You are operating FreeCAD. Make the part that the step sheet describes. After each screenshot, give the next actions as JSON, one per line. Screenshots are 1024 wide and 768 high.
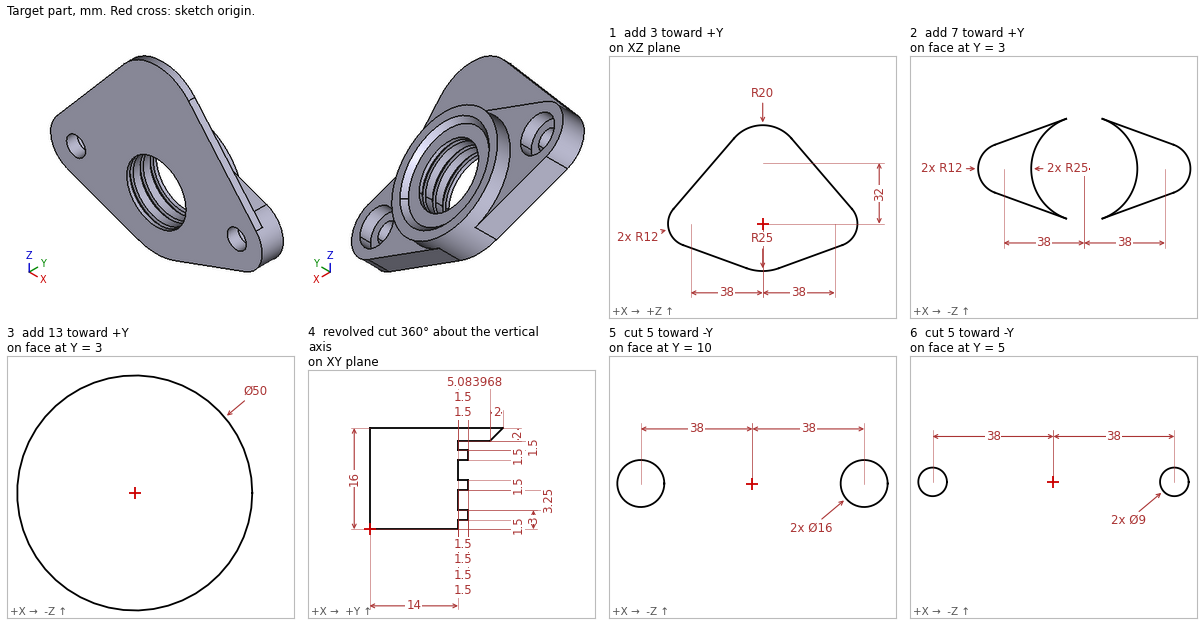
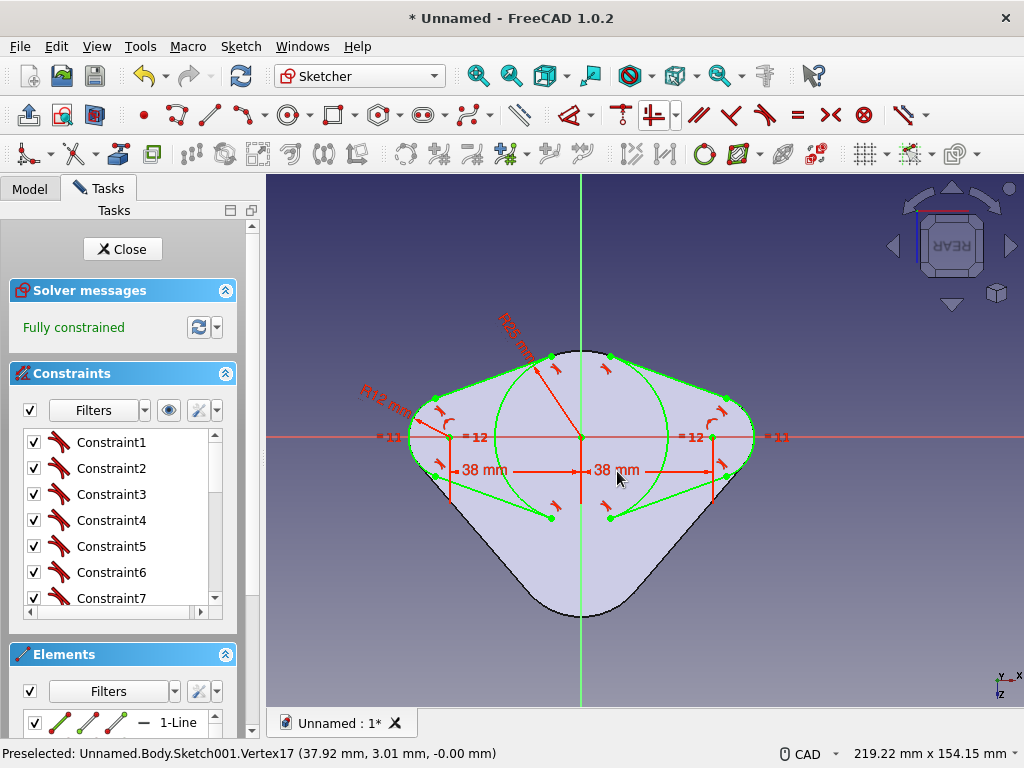
{"action": "left_click", "coordinate": [123, 249]}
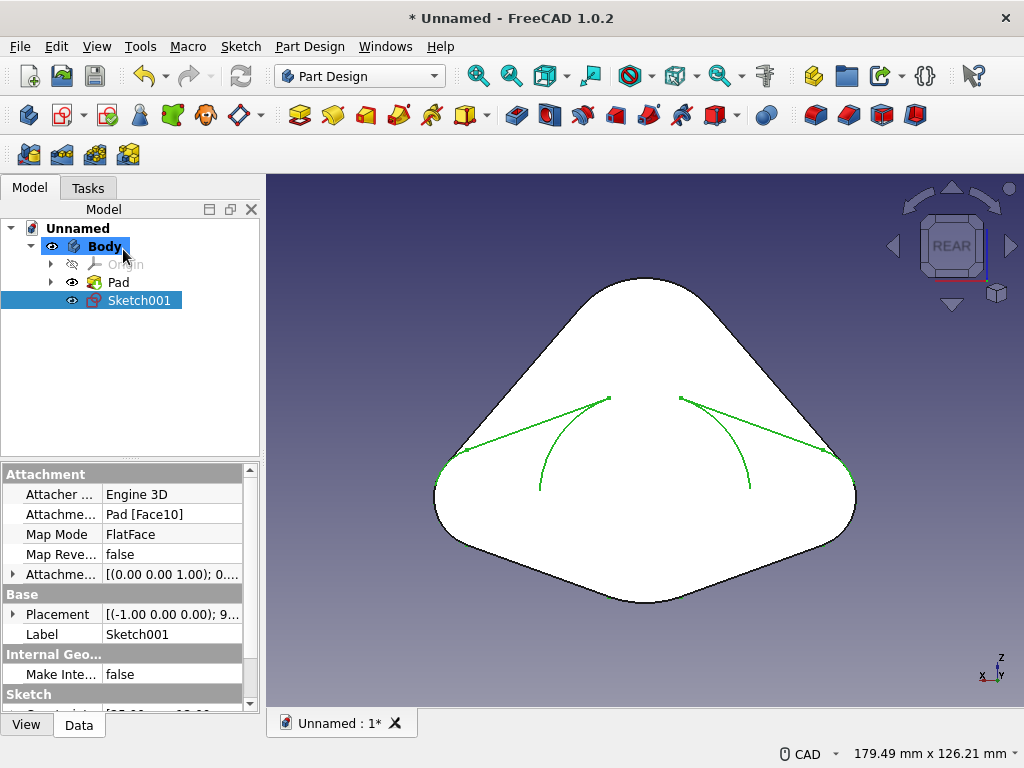
{"action": "left_click", "coordinate": [300, 116]}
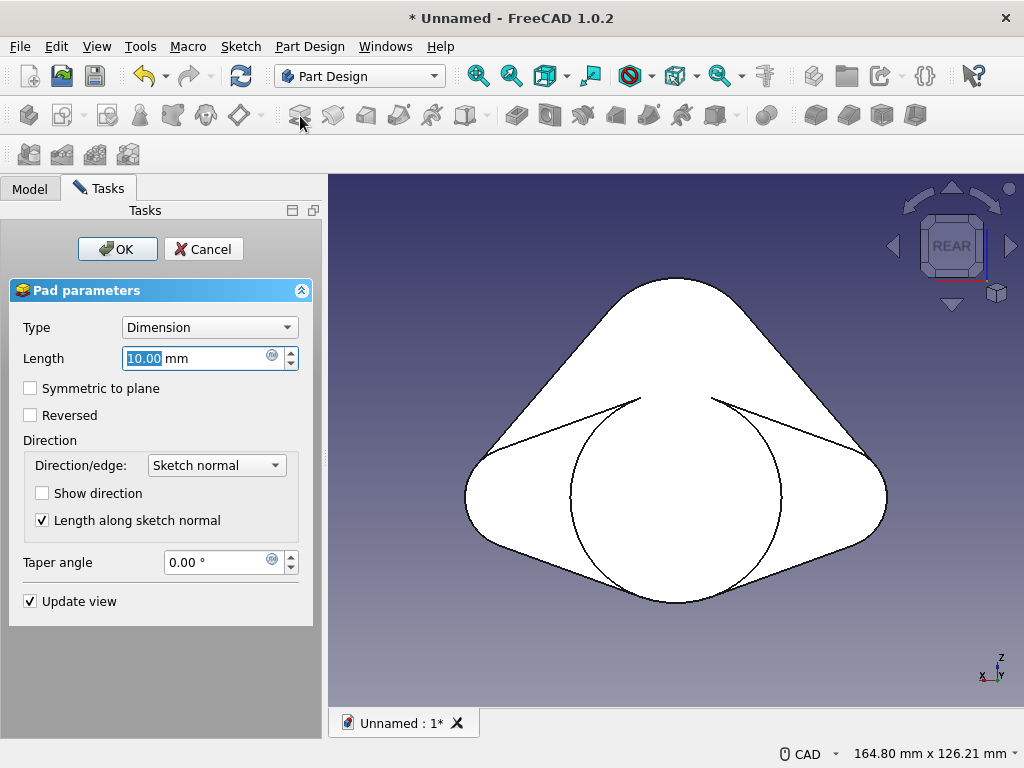
{"action": "type", "text": "7"}
{"action": "key", "text": "Tab"}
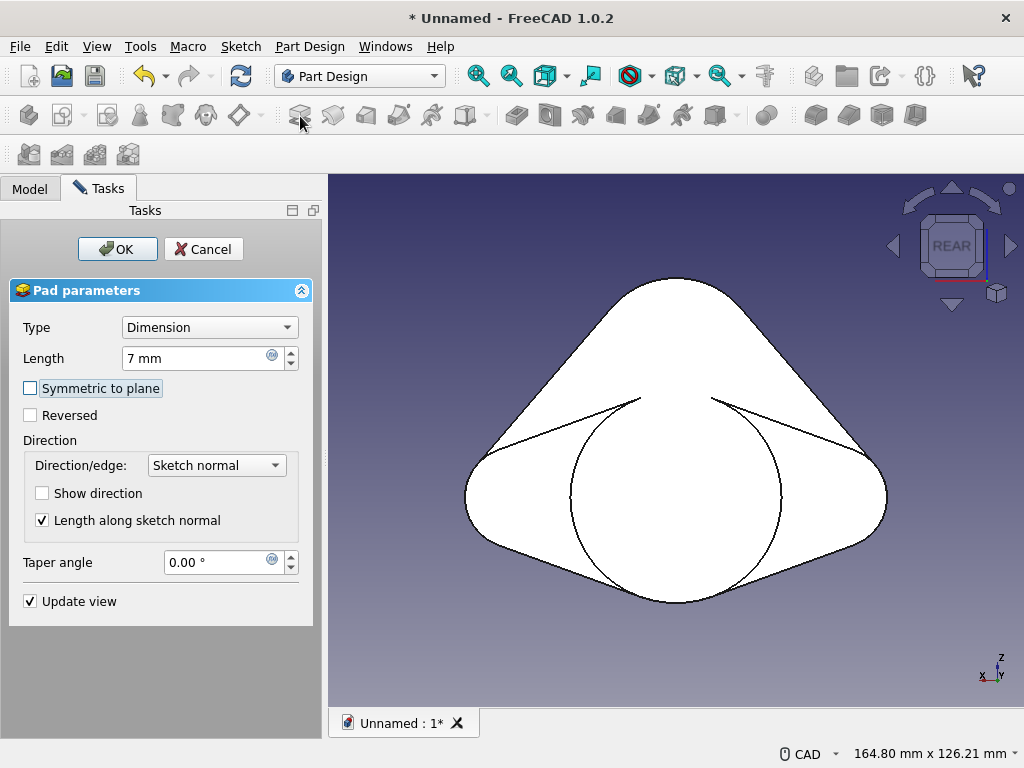
{"action": "left_click", "coordinate": [118, 249]}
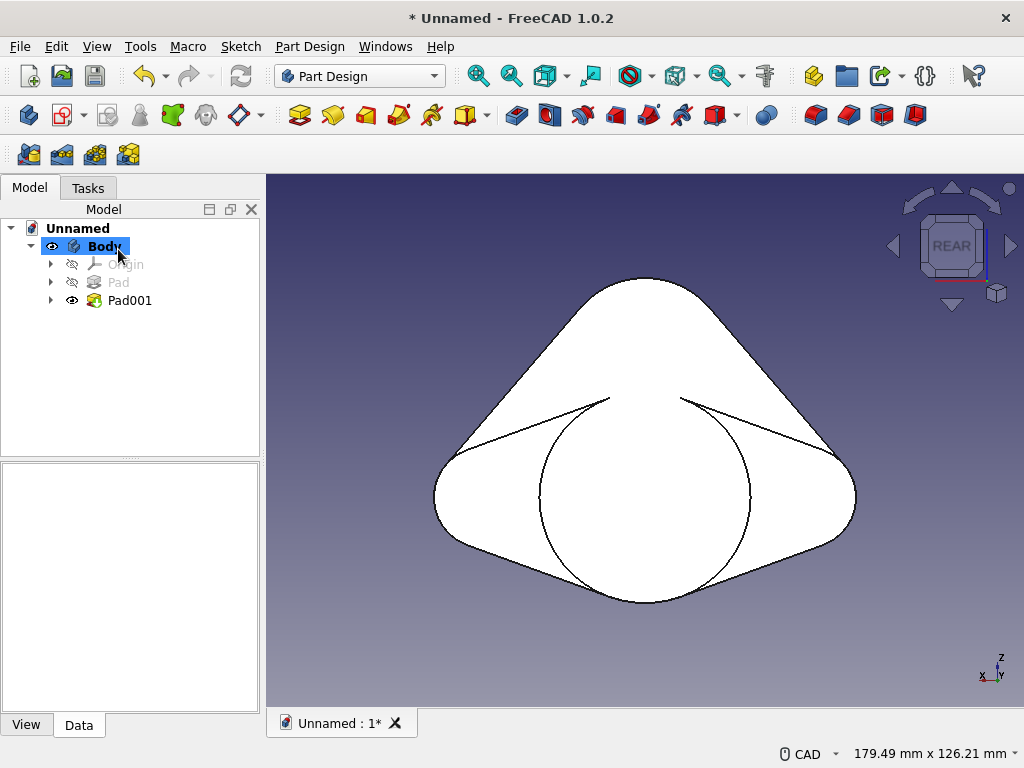
{"action": "left_click", "coordinate": [645, 486]}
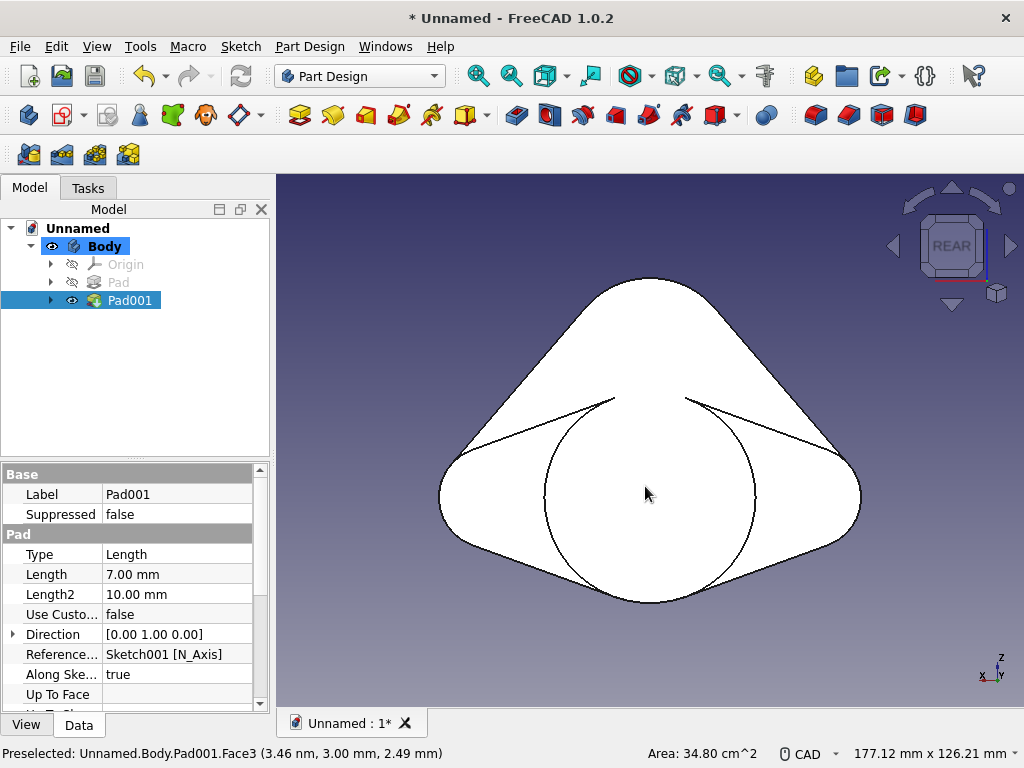
{"action": "left_click", "coordinate": [62, 116]}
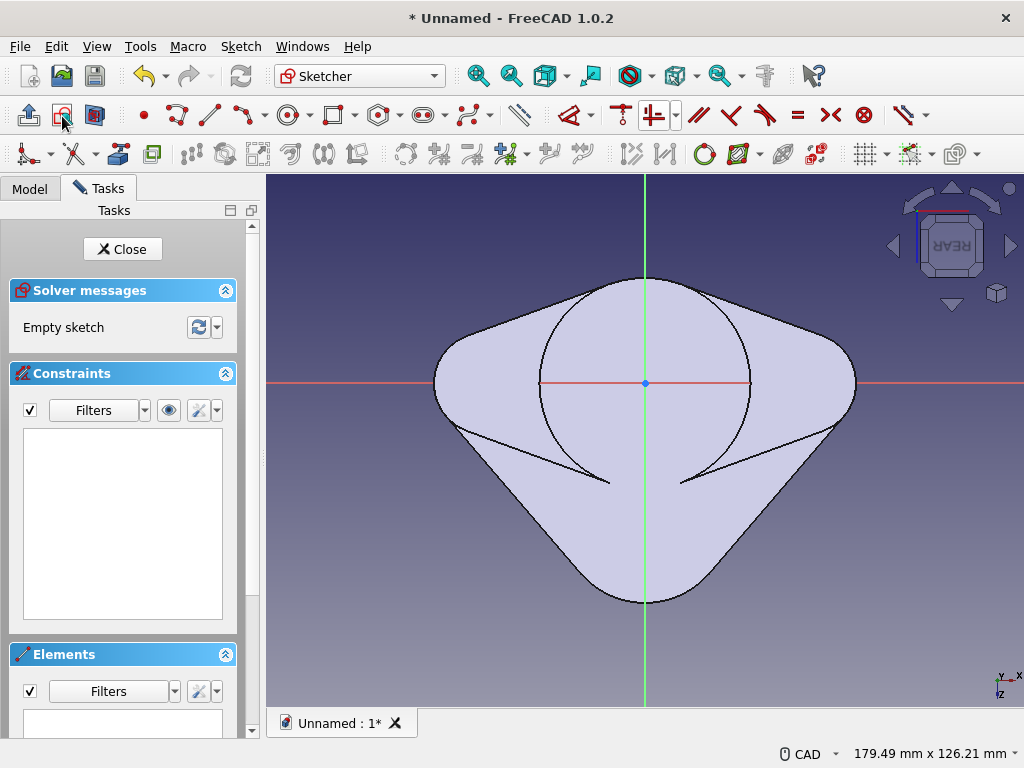
{"action": "scroll", "coordinate": [784, 268], "scroll_direction": "up", "scroll_amount": 2}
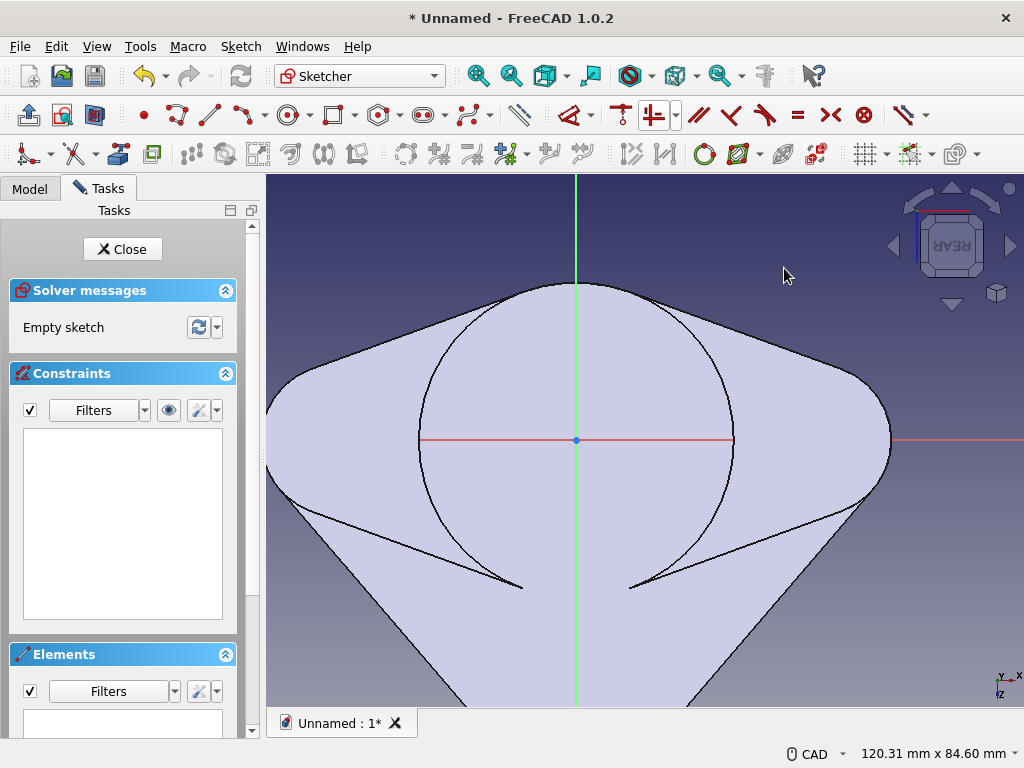
{"action": "left_click", "coordinate": [288, 116]}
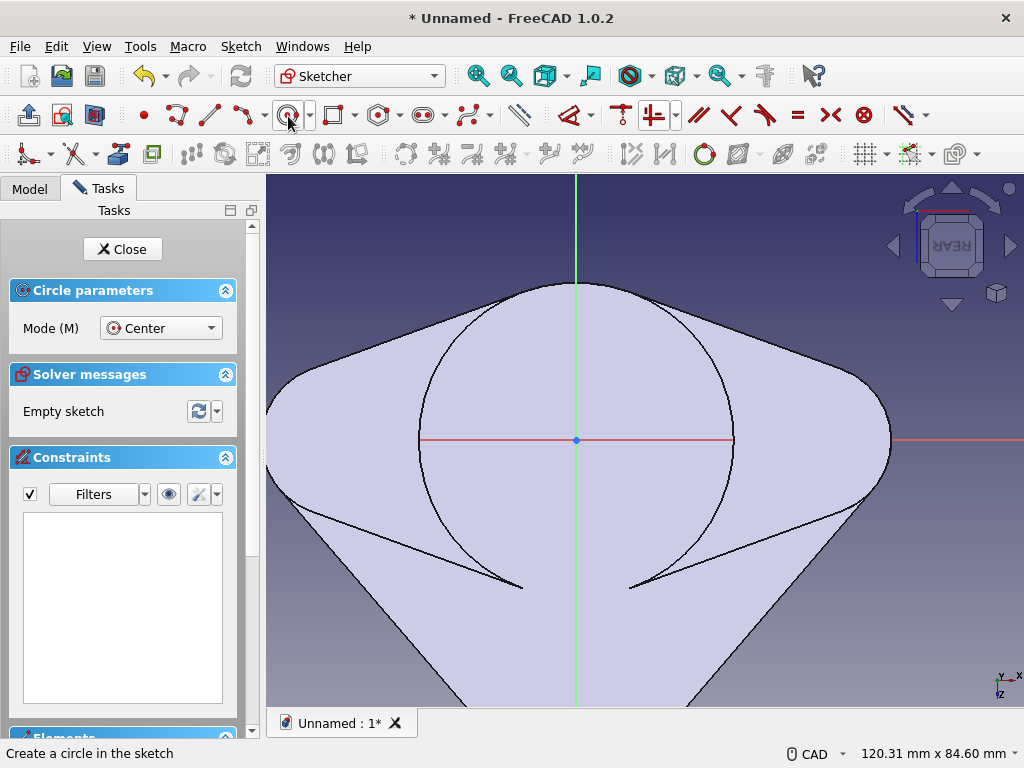
{"action": "left_click", "coordinate": [576, 440]}
{"action": "left_click", "coordinate": [688, 329]}
{"action": "key", "text": "Escape"}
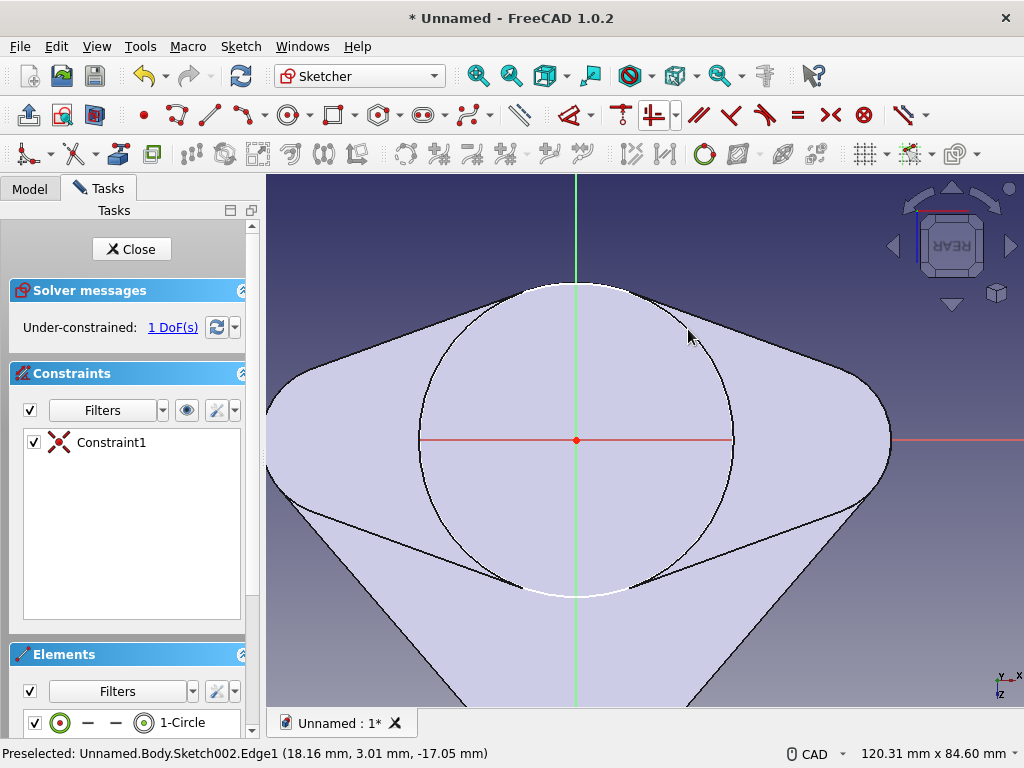
{"action": "left_click", "coordinate": [568, 116]}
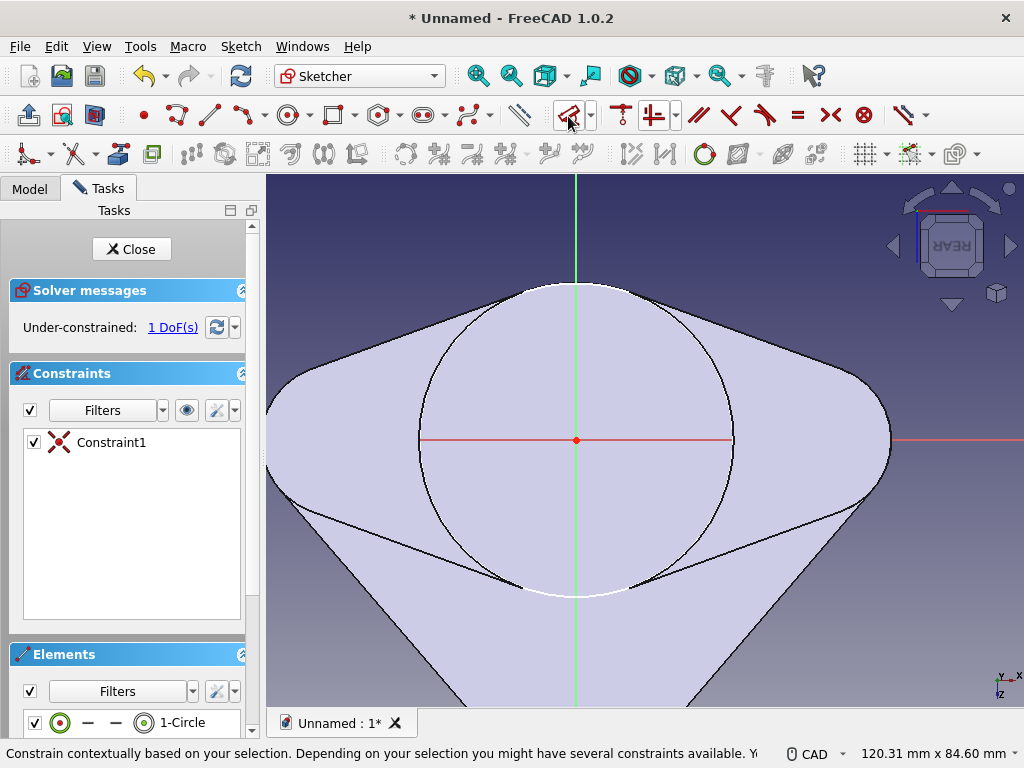
{"action": "left_click", "coordinate": [687, 329]}
{"action": "left_click", "coordinate": [710, 306]}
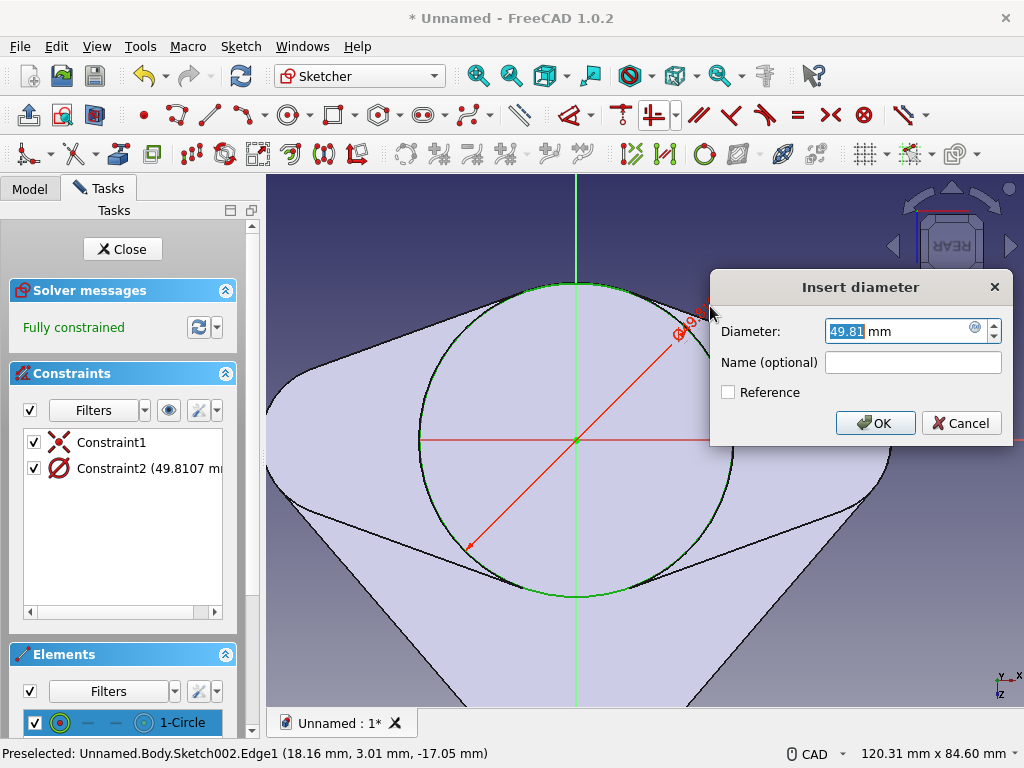
{"action": "type", "text": "50"}
{"action": "key", "text": "Return"}
{"action": "key", "text": "Escape"}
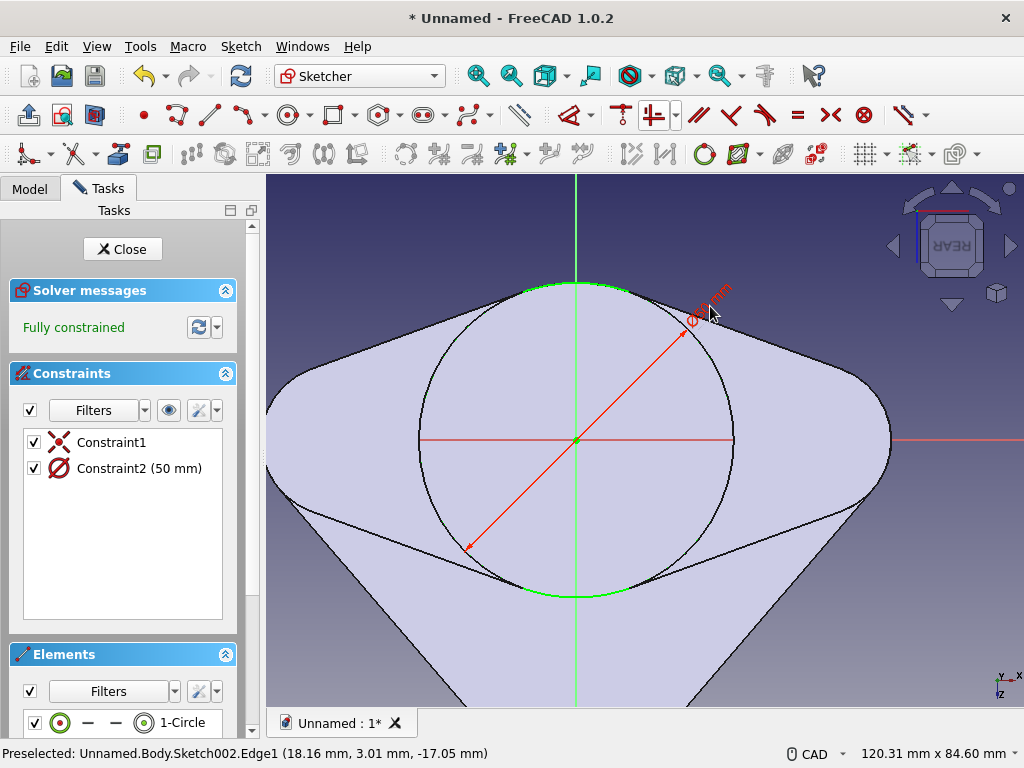
{"action": "left_click", "coordinate": [123, 249]}